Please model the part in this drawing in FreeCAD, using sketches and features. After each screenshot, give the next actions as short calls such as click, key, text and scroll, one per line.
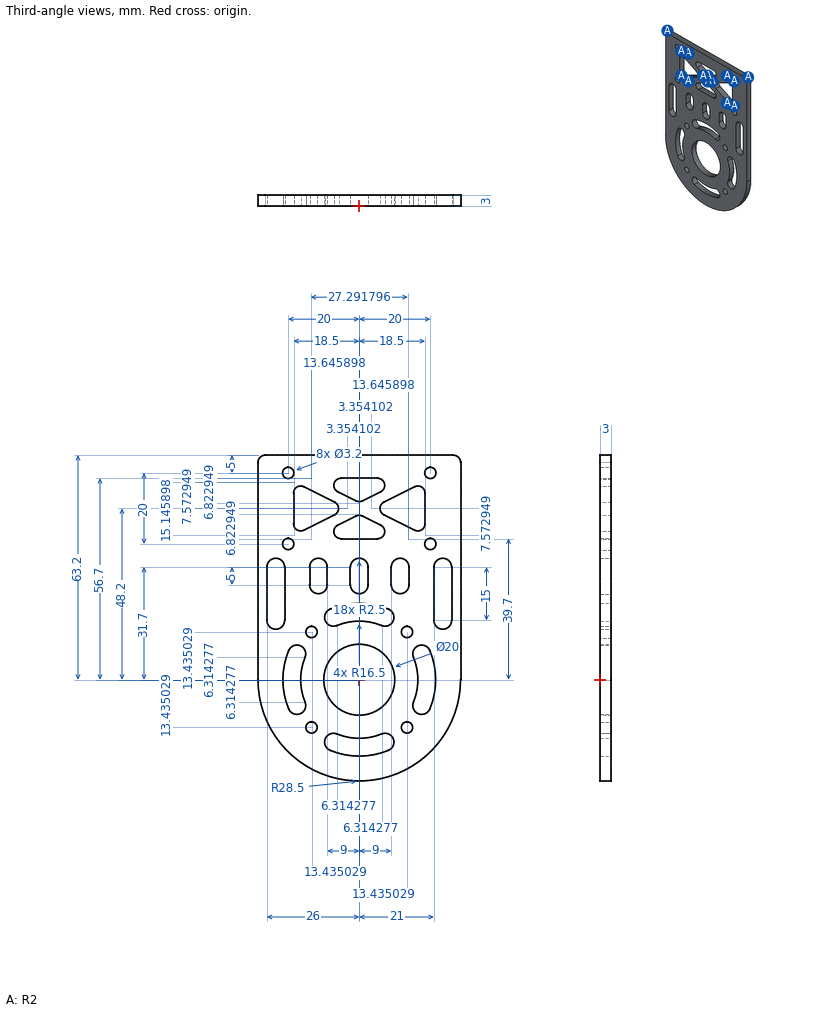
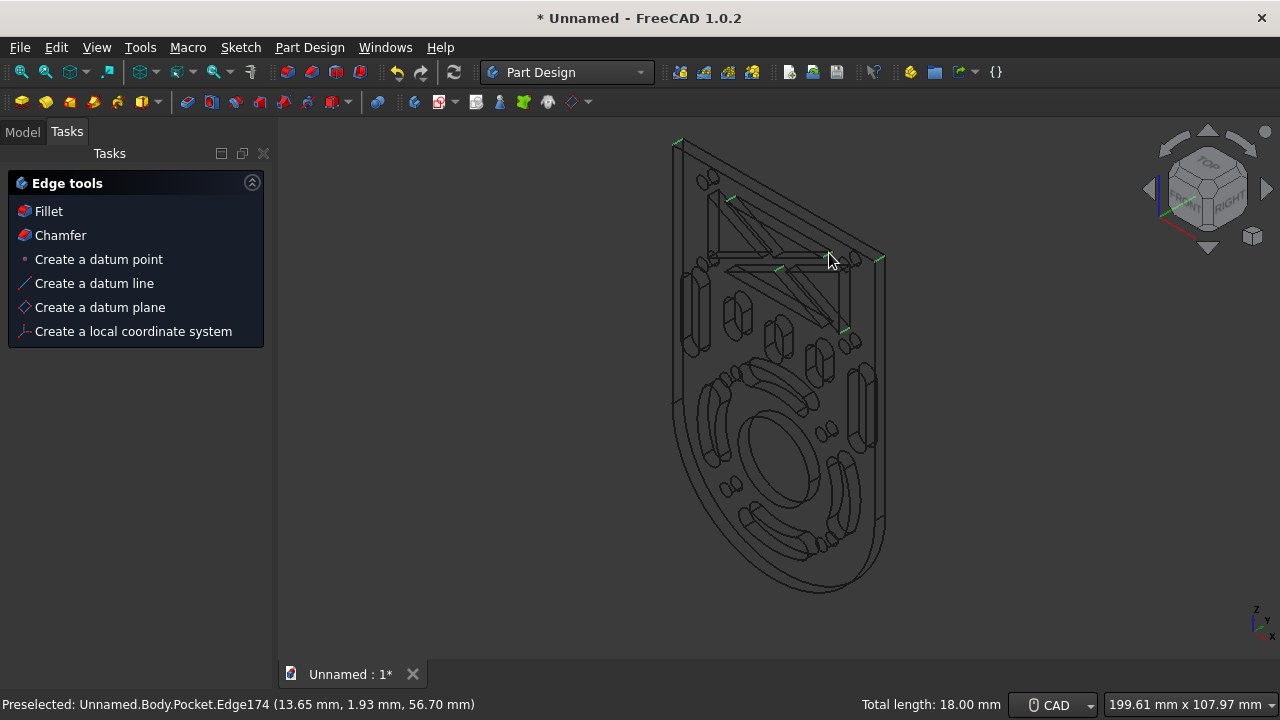
click(714, 191, ctrl)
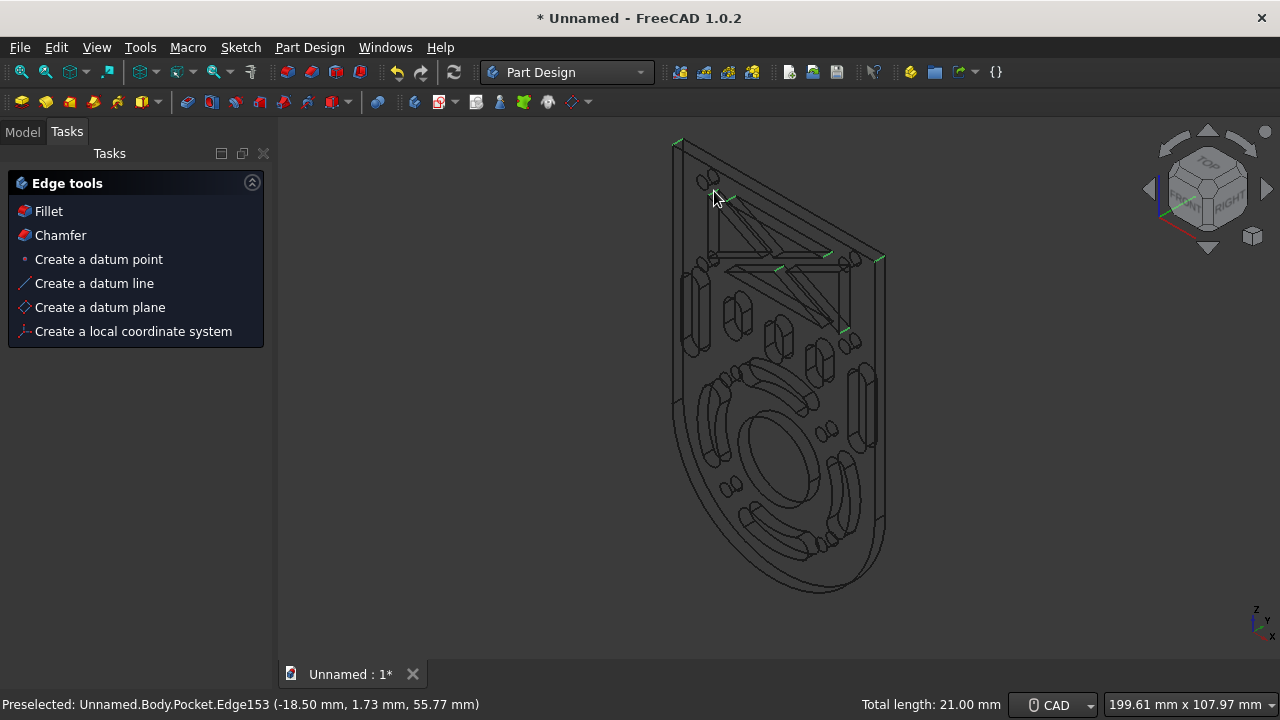
scroll(791, 268, up, 5)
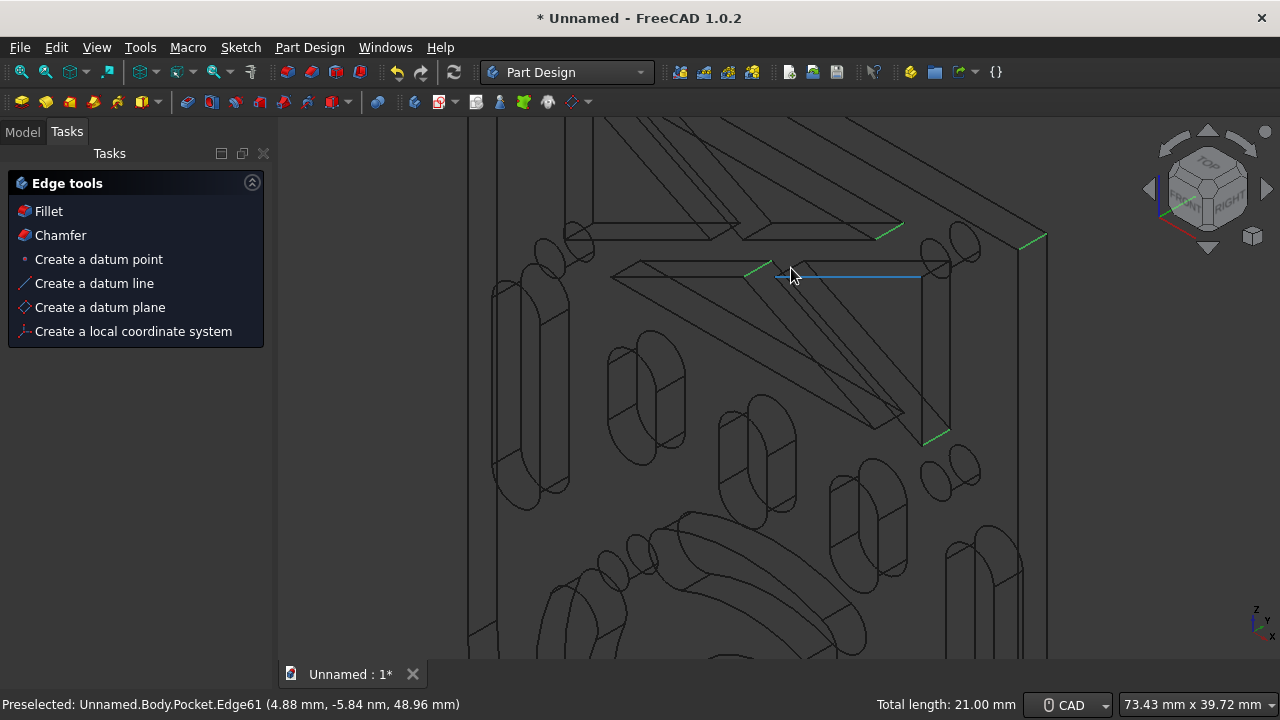
click(790, 268, ctrl)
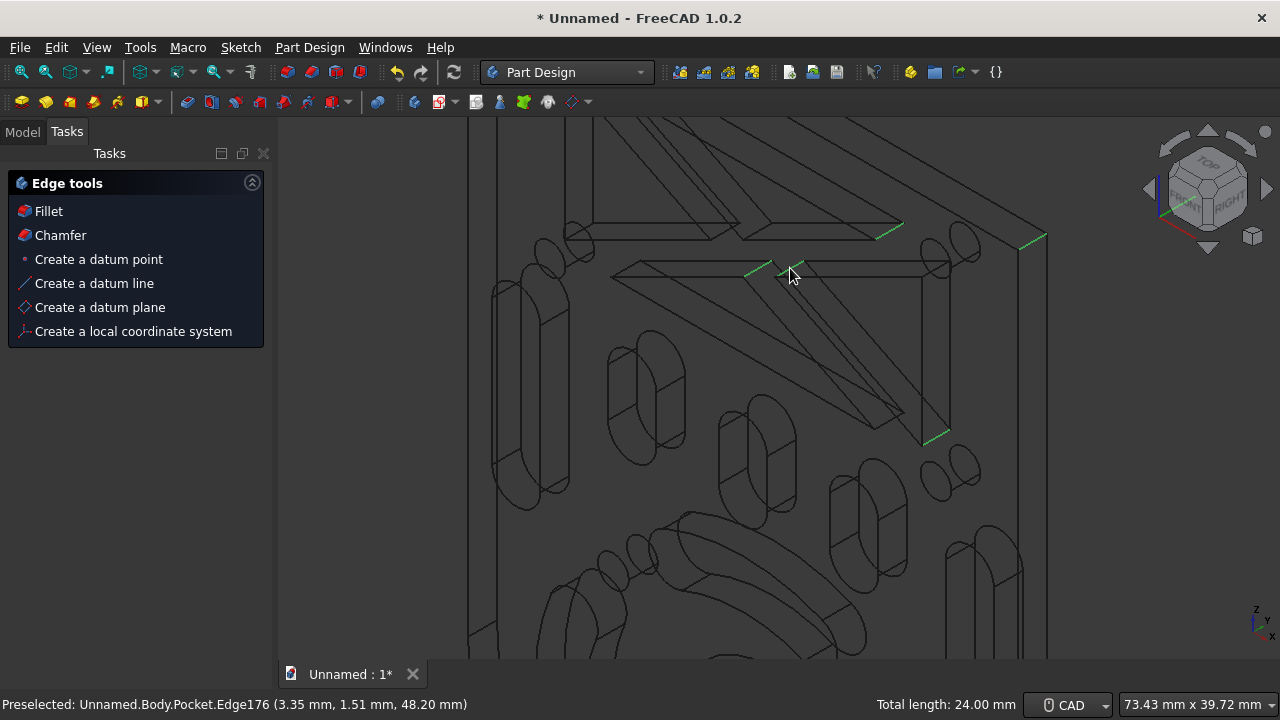
click(939, 266, ctrl)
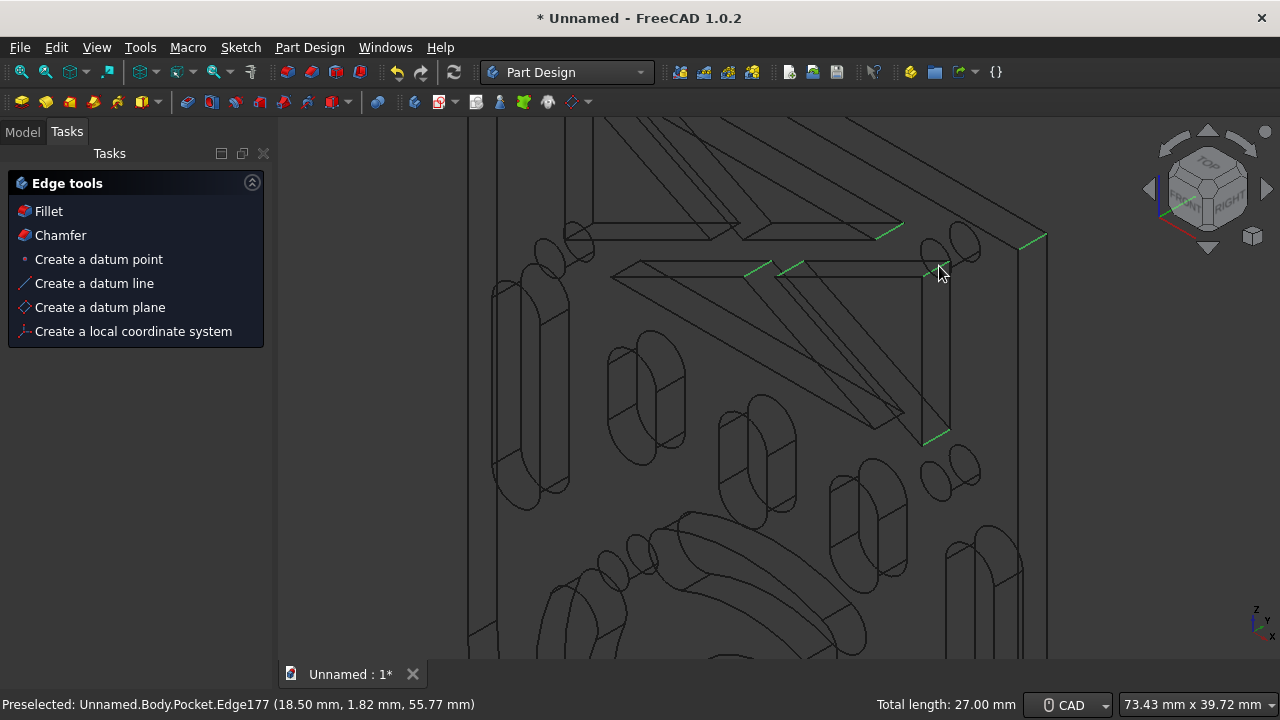
click(626, 268, ctrl)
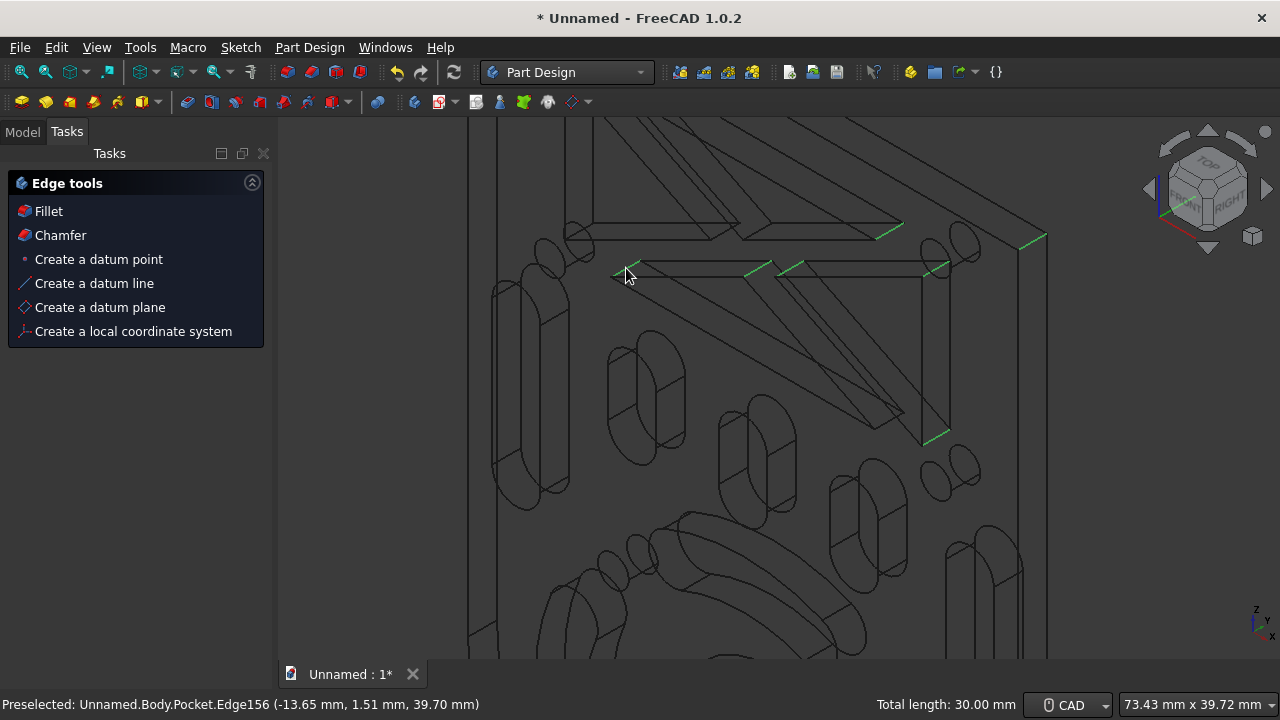
click(889, 420, ctrl)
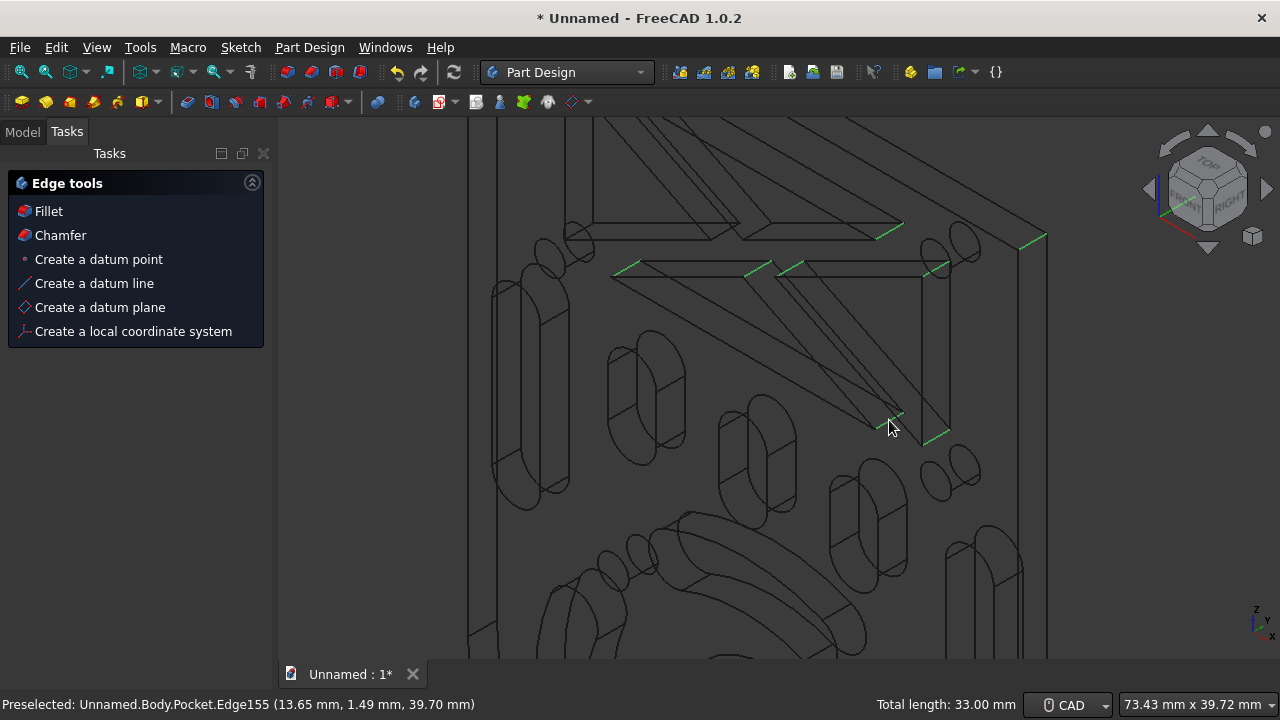
click(757, 231, ctrl)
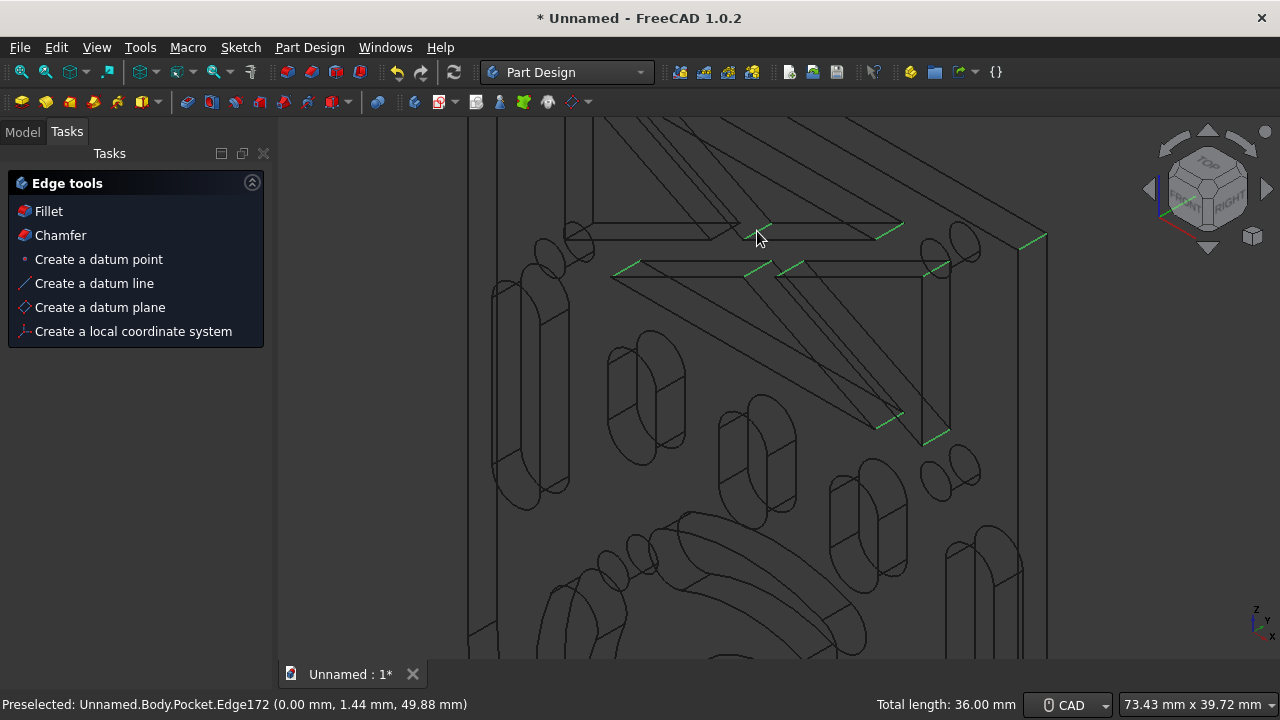
click(579, 231, ctrl)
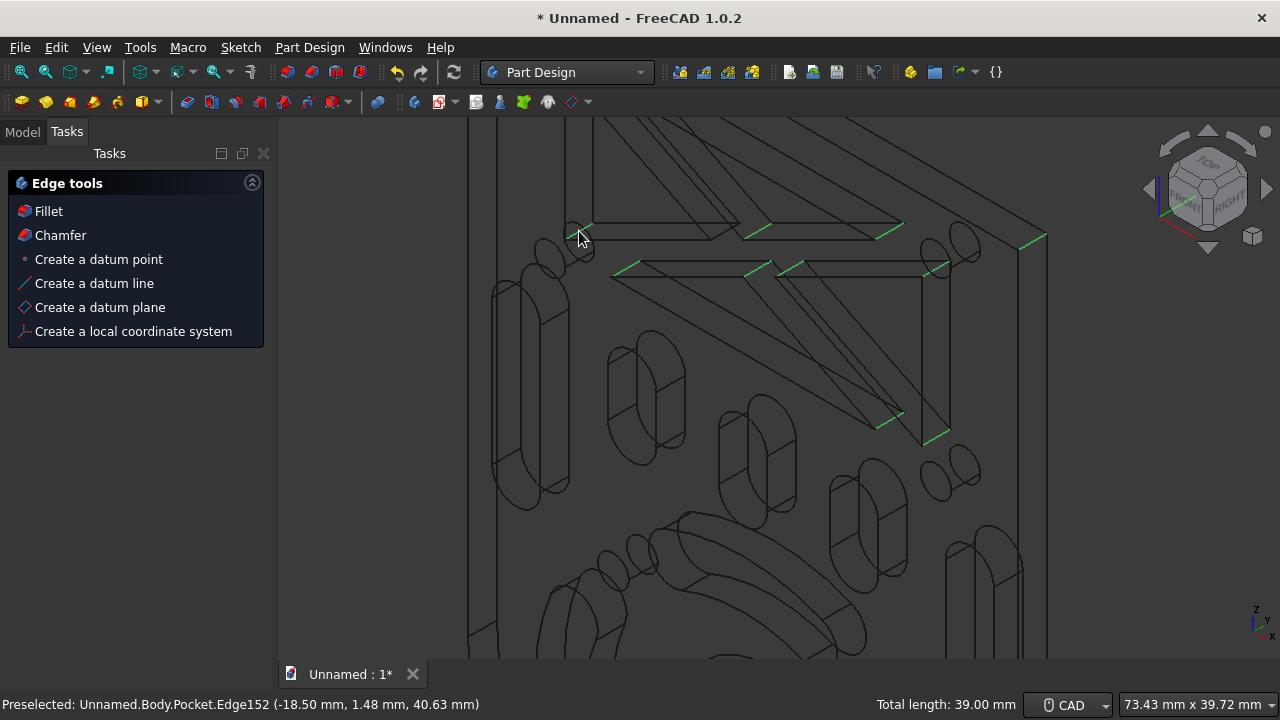
click(725, 231, ctrl)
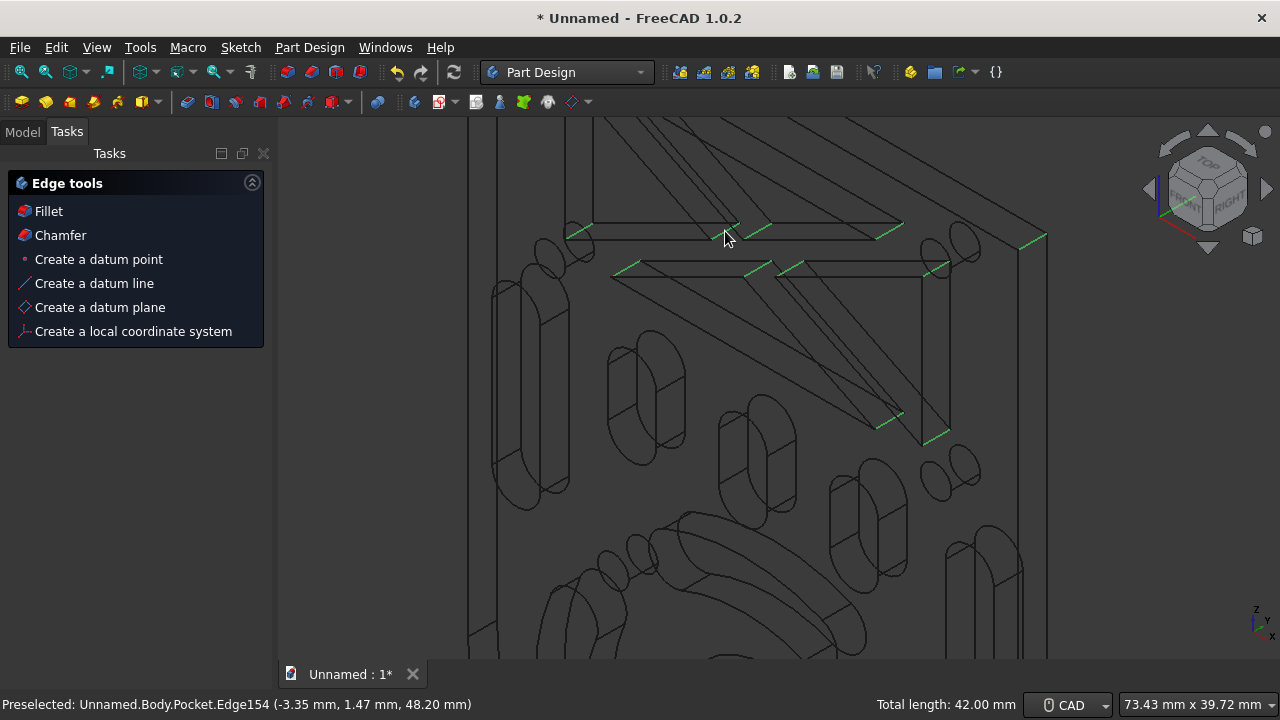
key(v)
key(1)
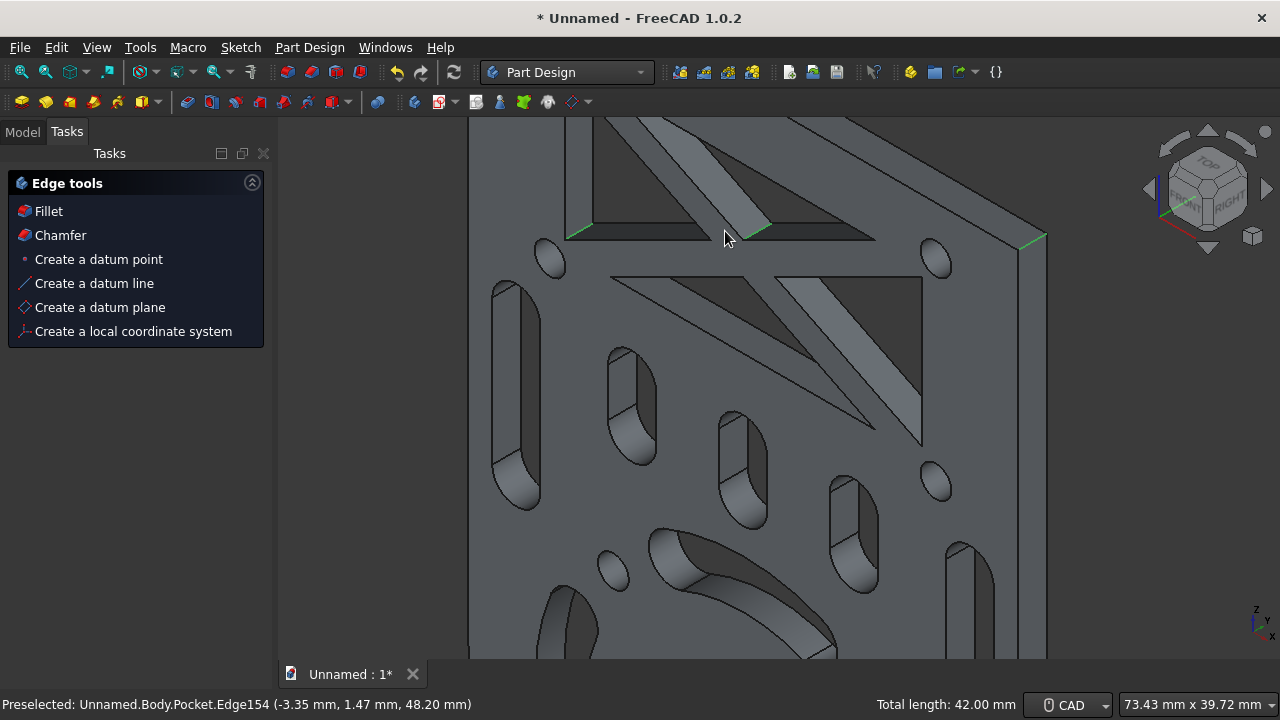
click(288, 72)